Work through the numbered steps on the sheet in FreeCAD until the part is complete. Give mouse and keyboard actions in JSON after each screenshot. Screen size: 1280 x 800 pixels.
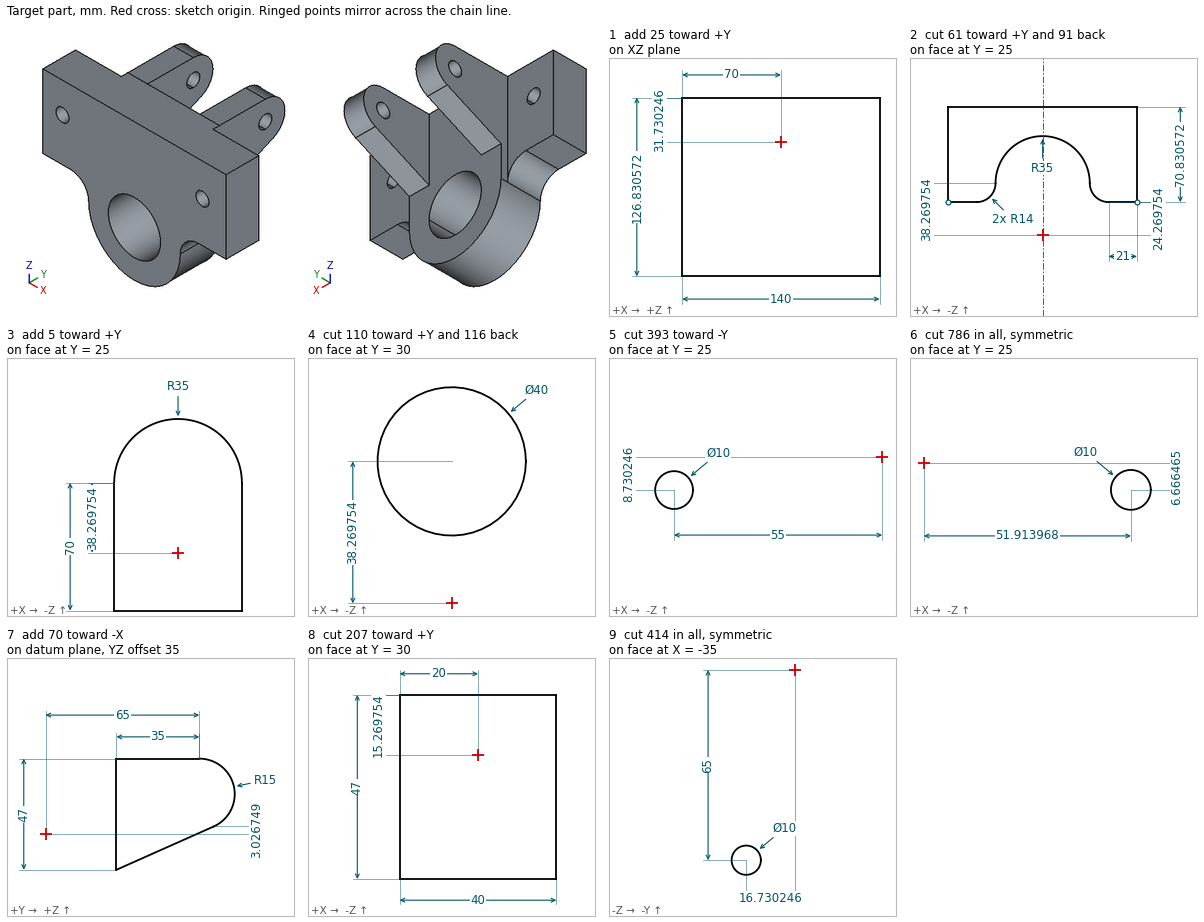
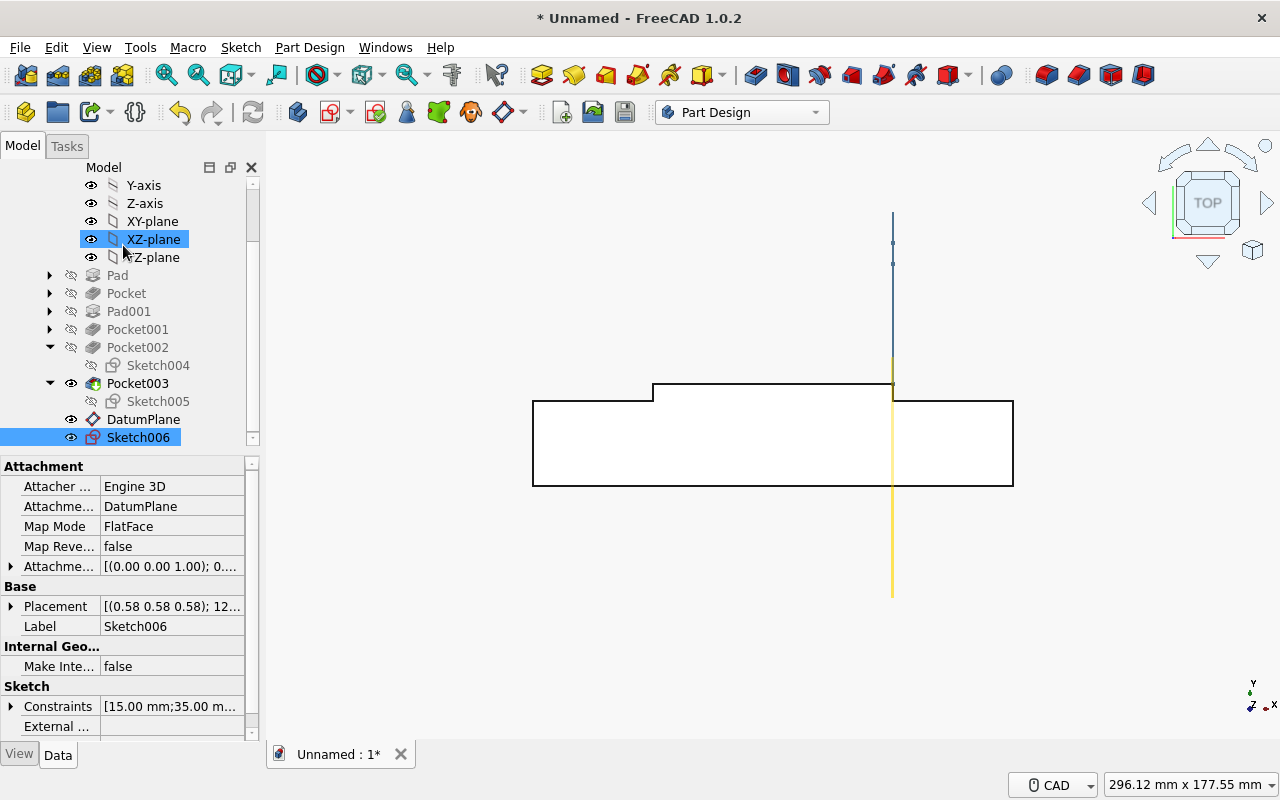
{"action": "left_click", "coordinate": [542, 76]}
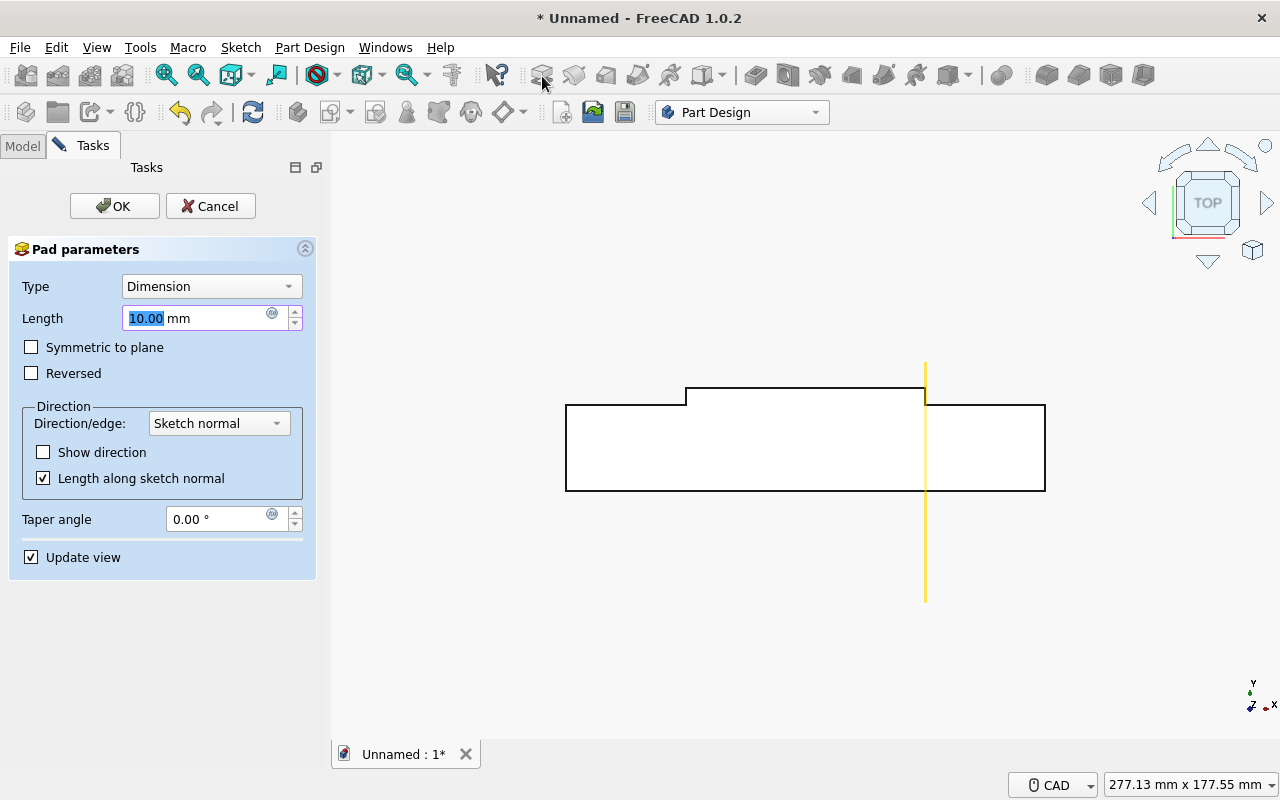
{"action": "type", "text": "70"}
{"action": "key", "text": "Tab"}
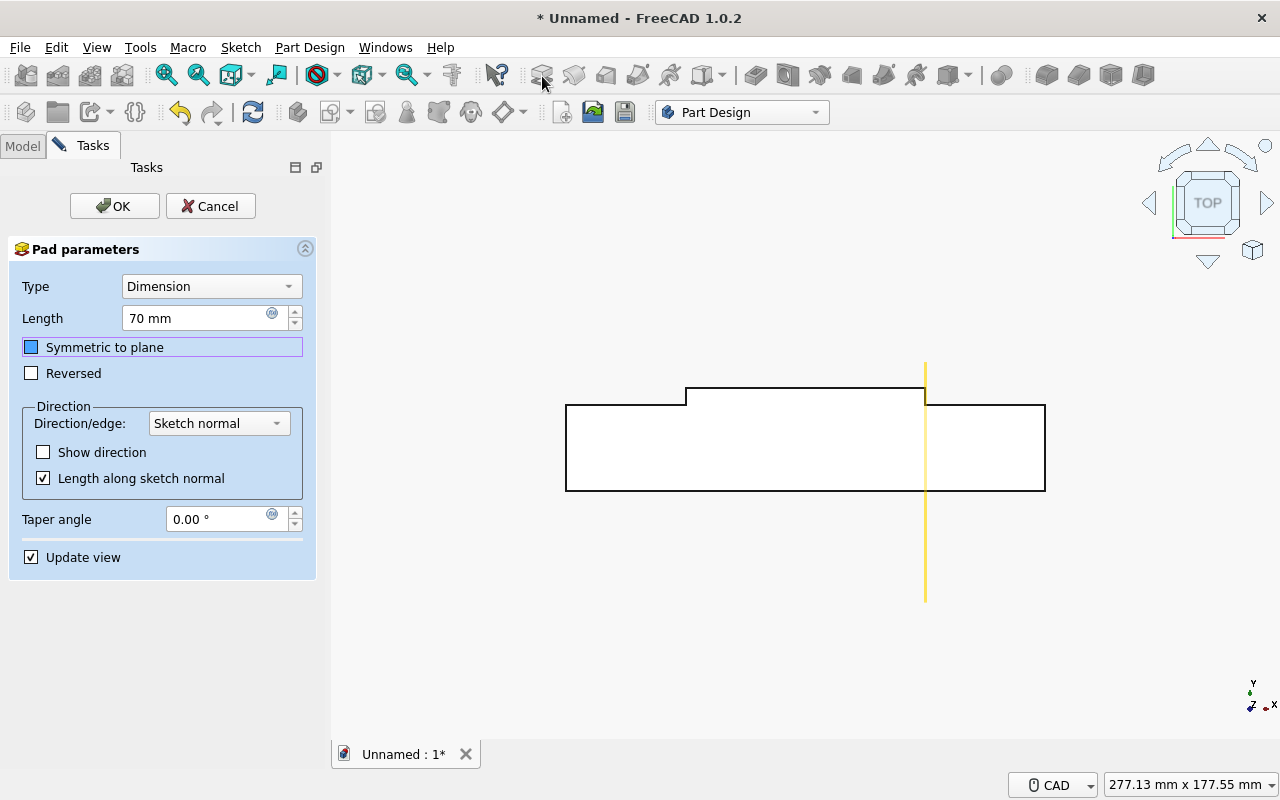
{"action": "left_click", "coordinate": [30, 373]}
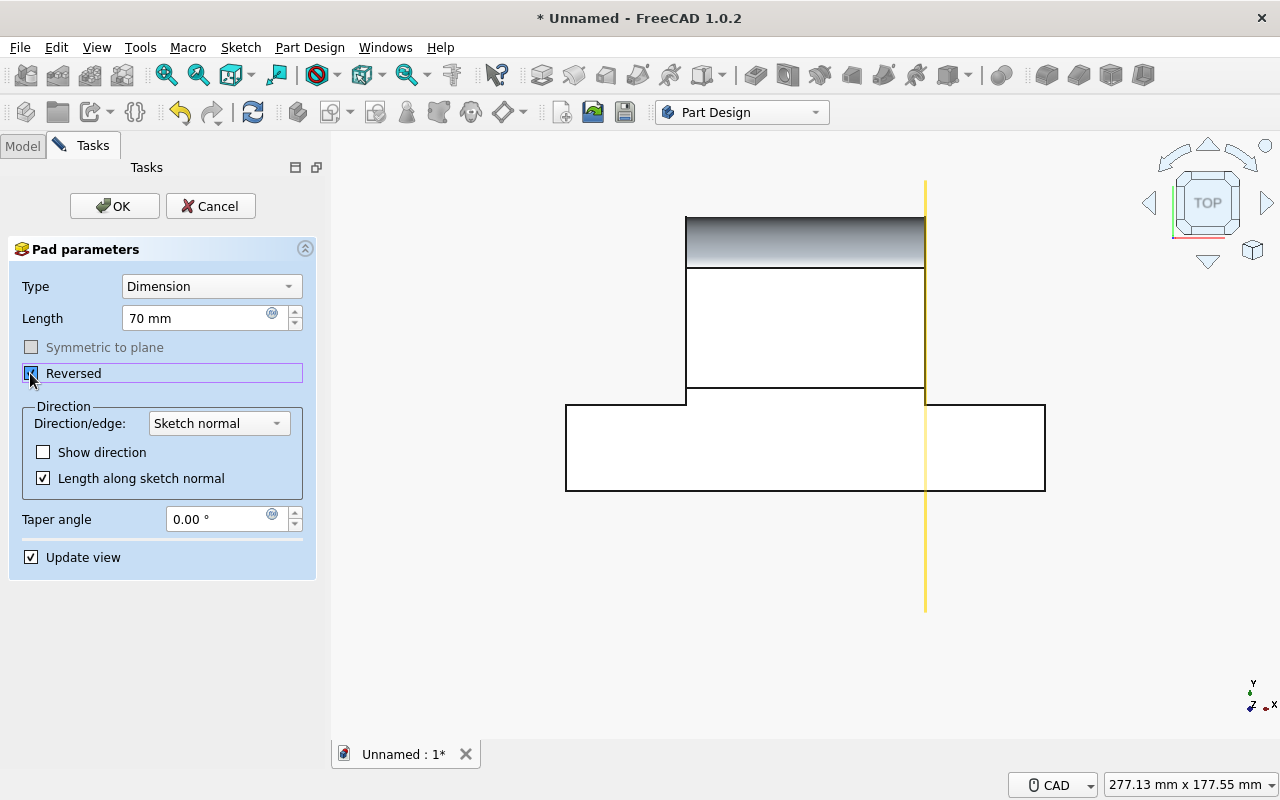
{"action": "left_click", "coordinate": [115, 206]}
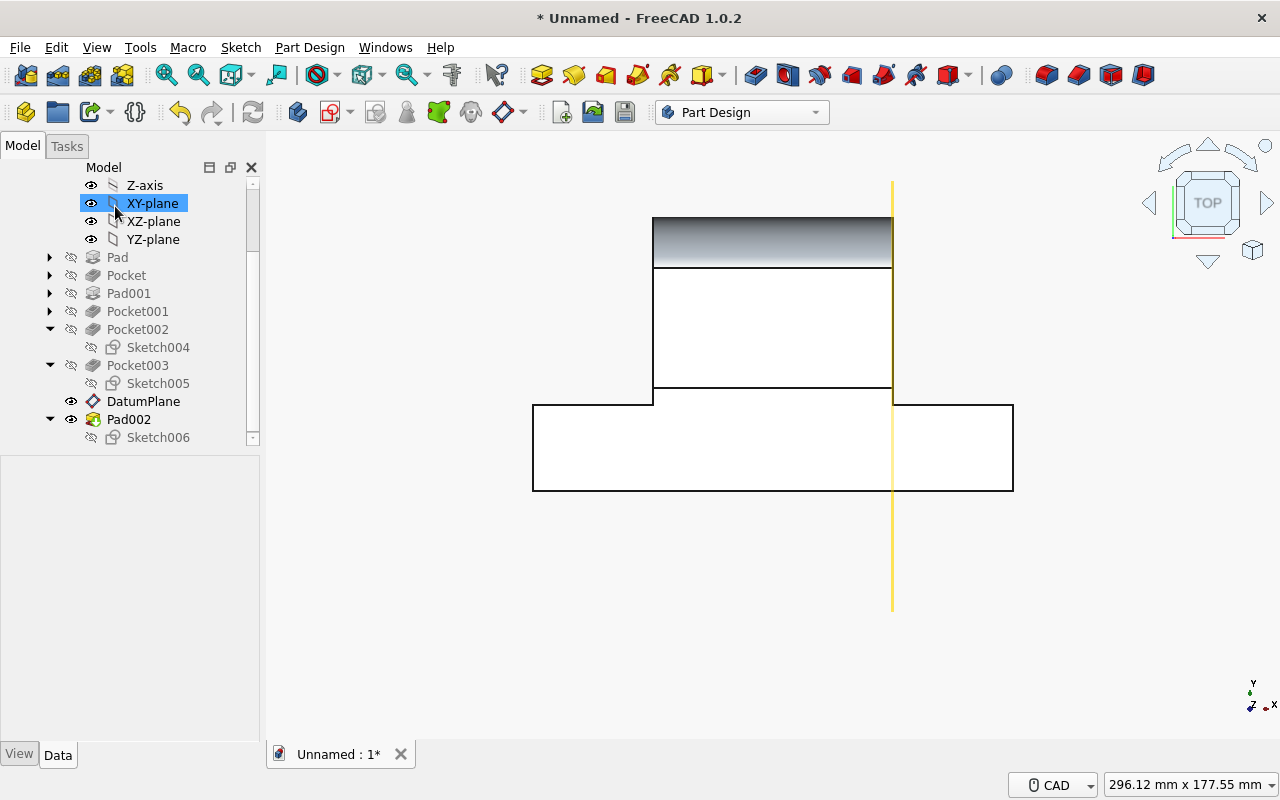
{"action": "left_click", "coordinate": [116, 401]}
{"action": "key", "text": "space"}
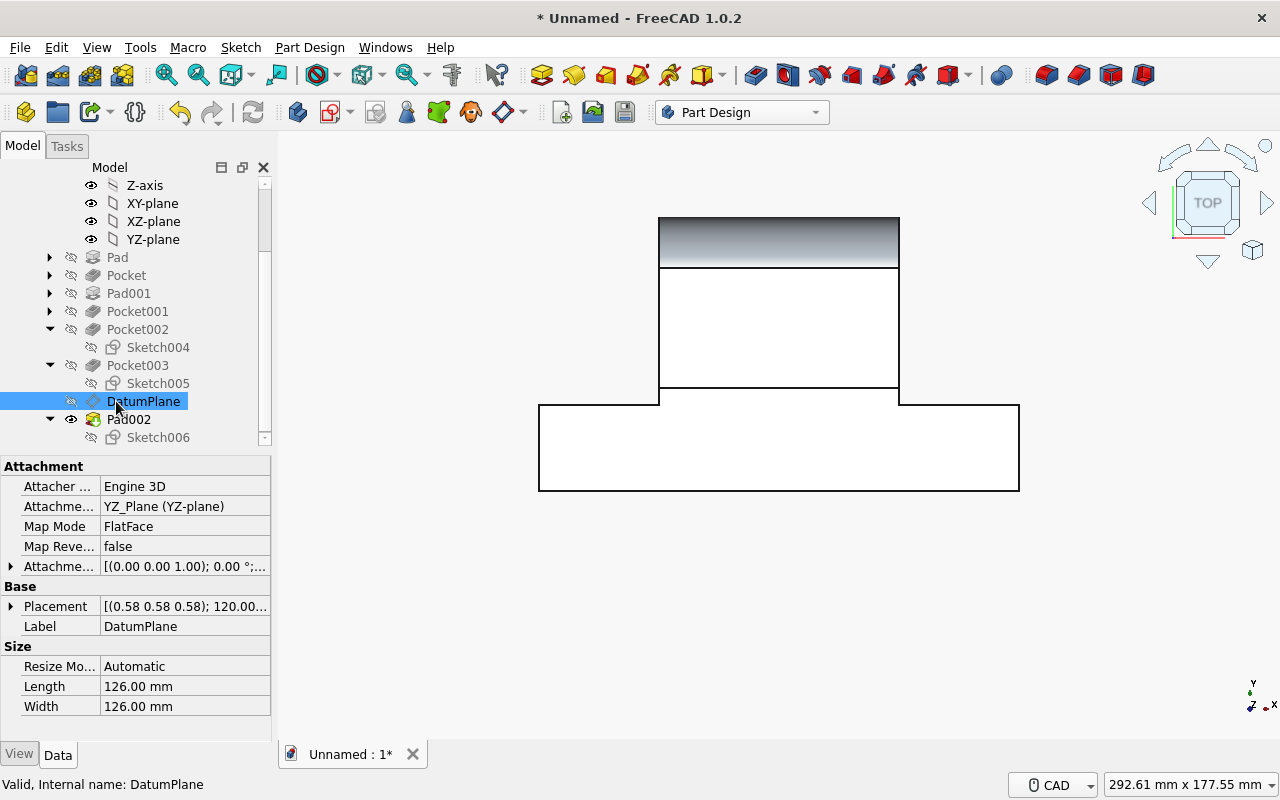
{"action": "key", "text": "4"}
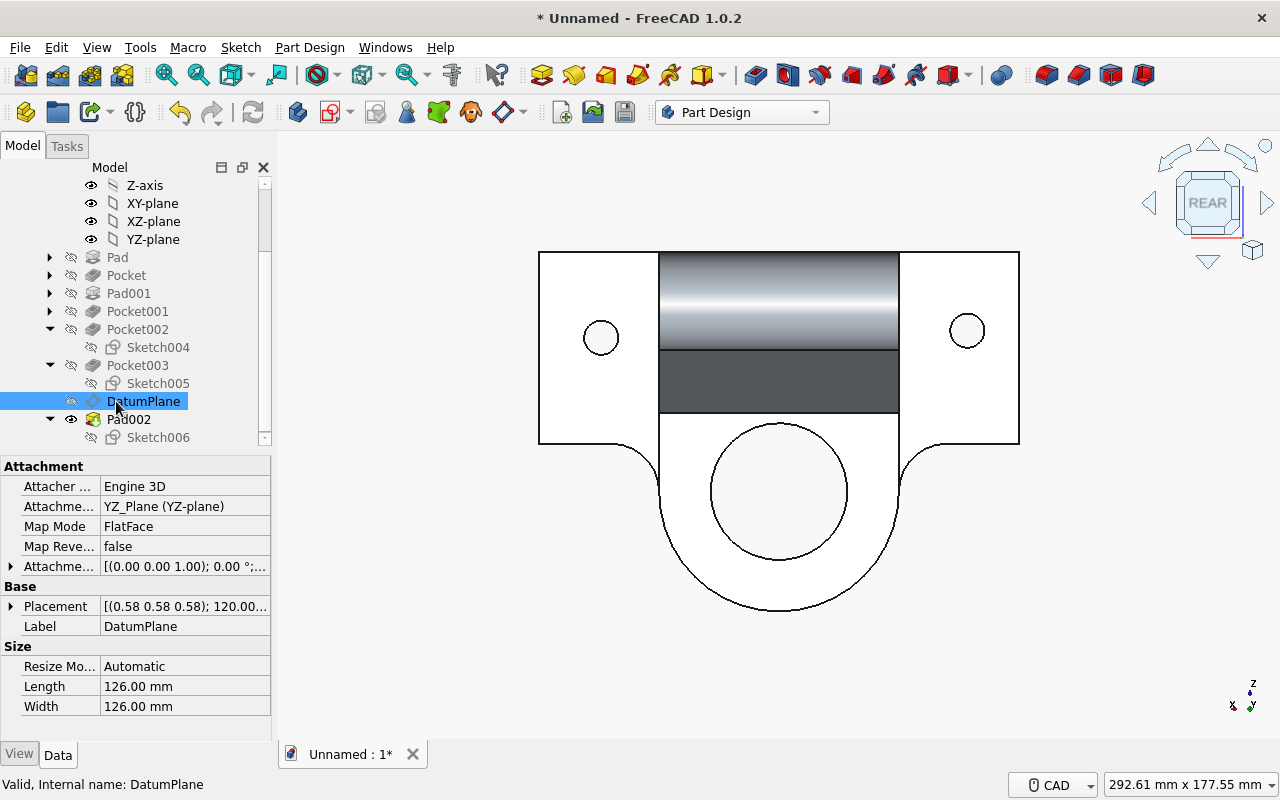
{"action": "left_click", "coordinate": [676, 454]}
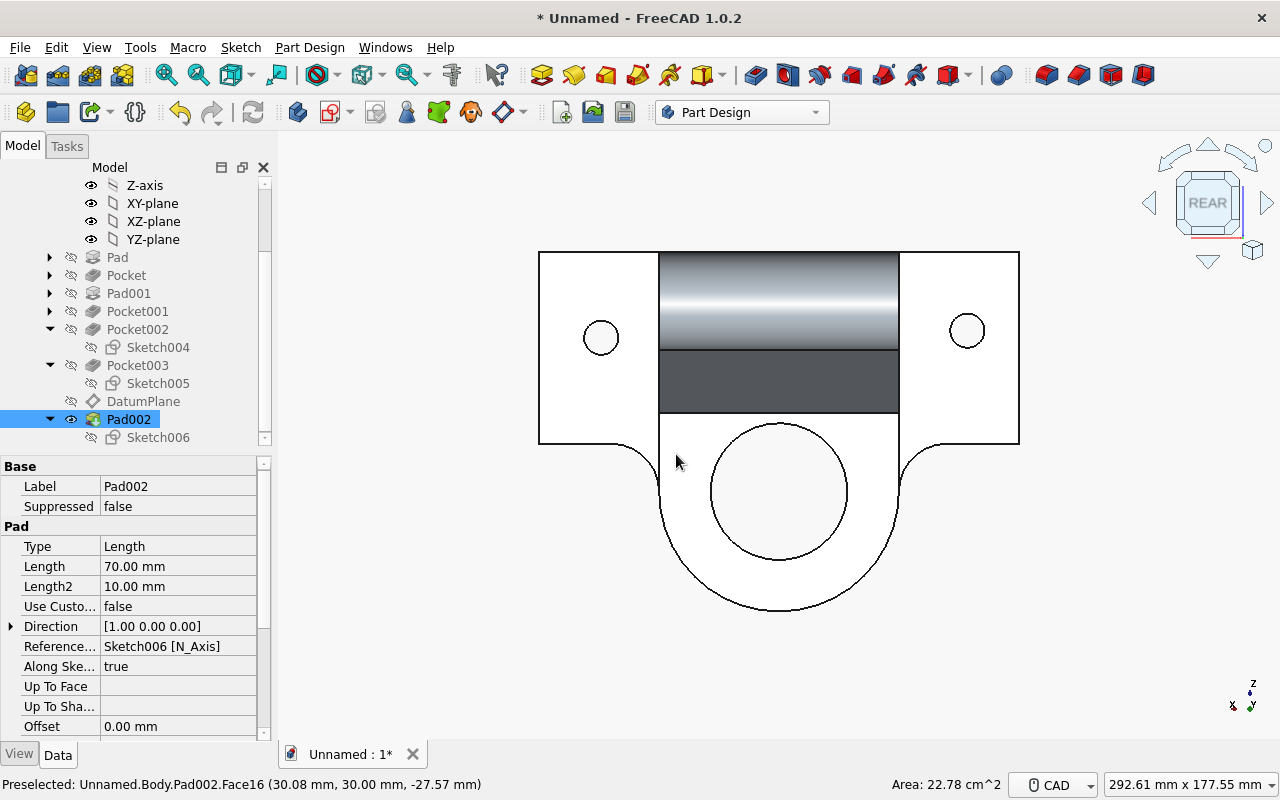
{"action": "left_click", "coordinate": [330, 112]}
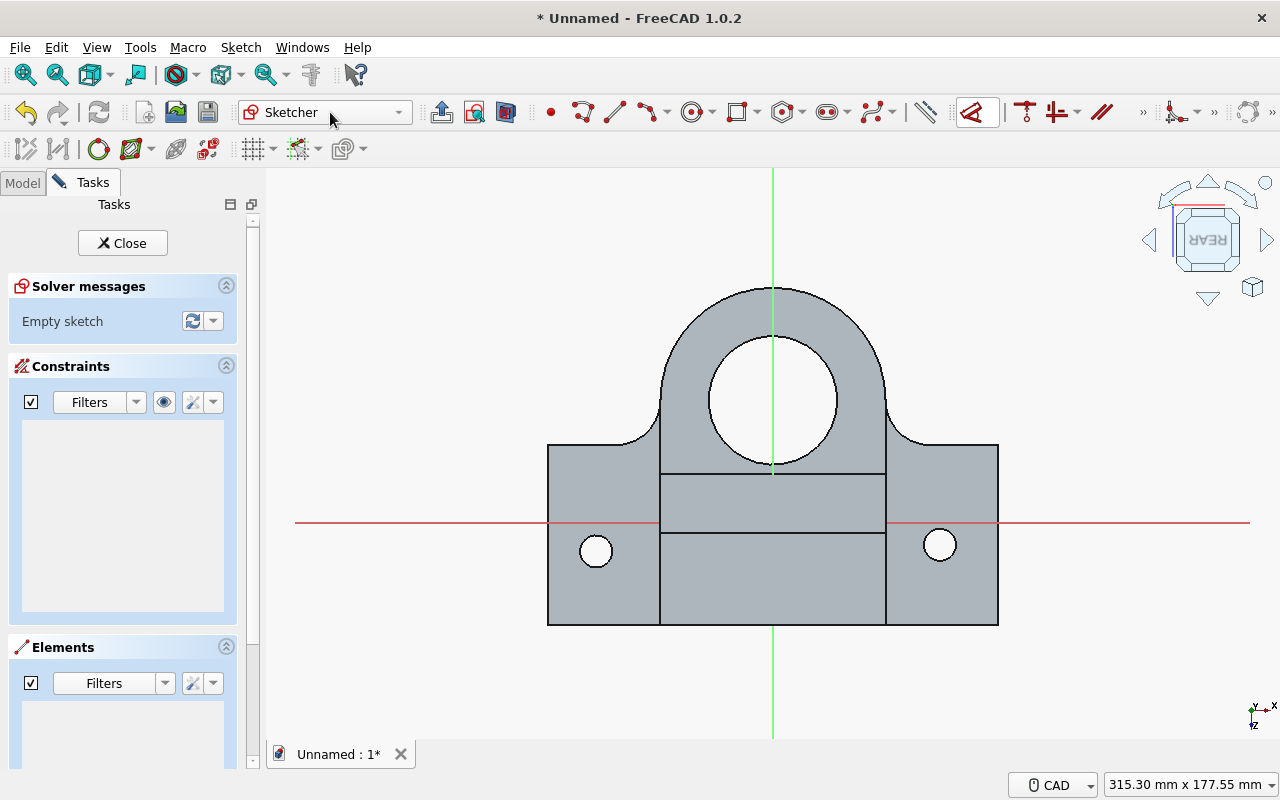
{"action": "scroll", "coordinate": [829, 628], "scroll_direction": "up", "scroll_amount": 4}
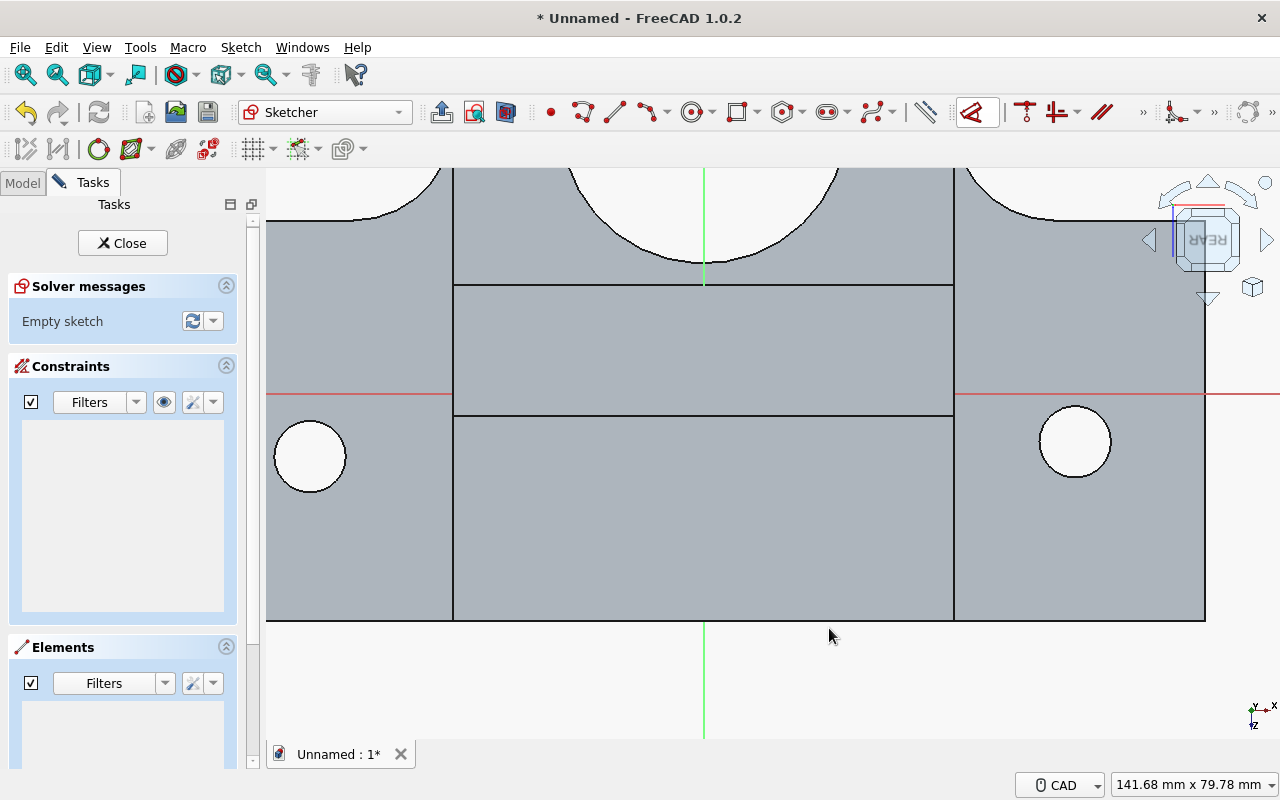
{"action": "left_click", "coordinate": [738, 112]}